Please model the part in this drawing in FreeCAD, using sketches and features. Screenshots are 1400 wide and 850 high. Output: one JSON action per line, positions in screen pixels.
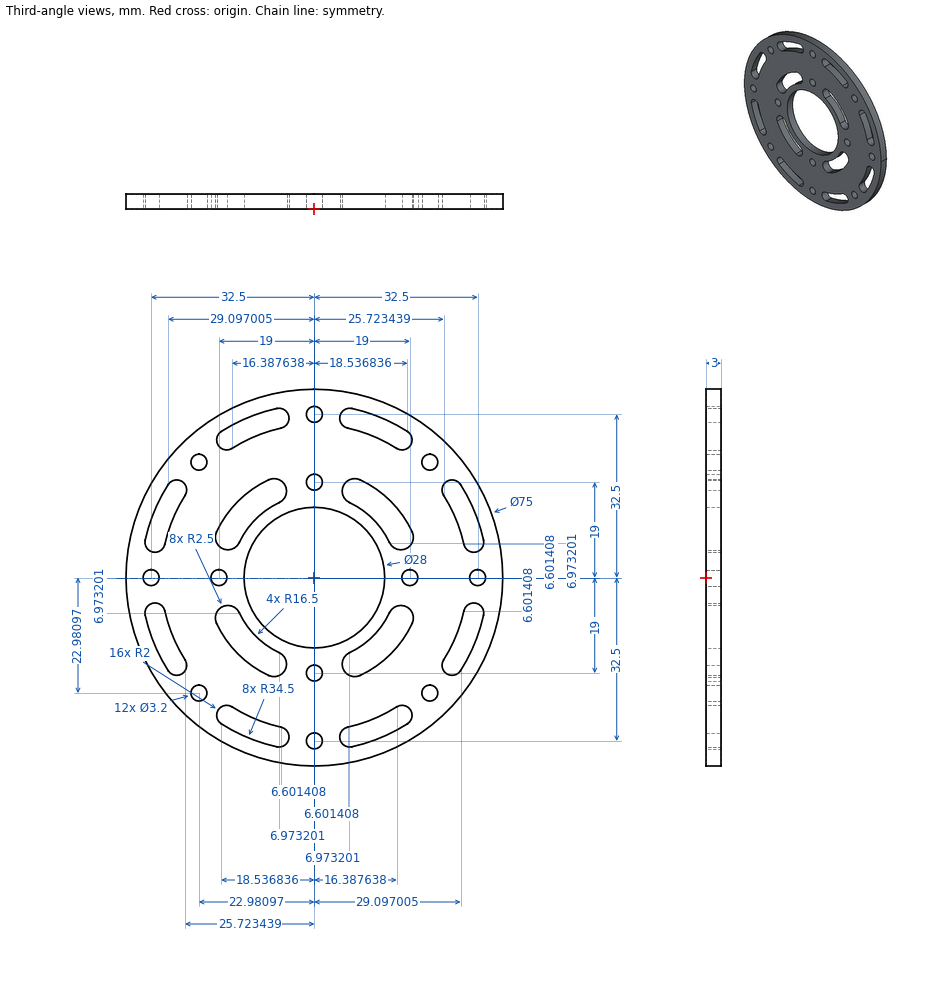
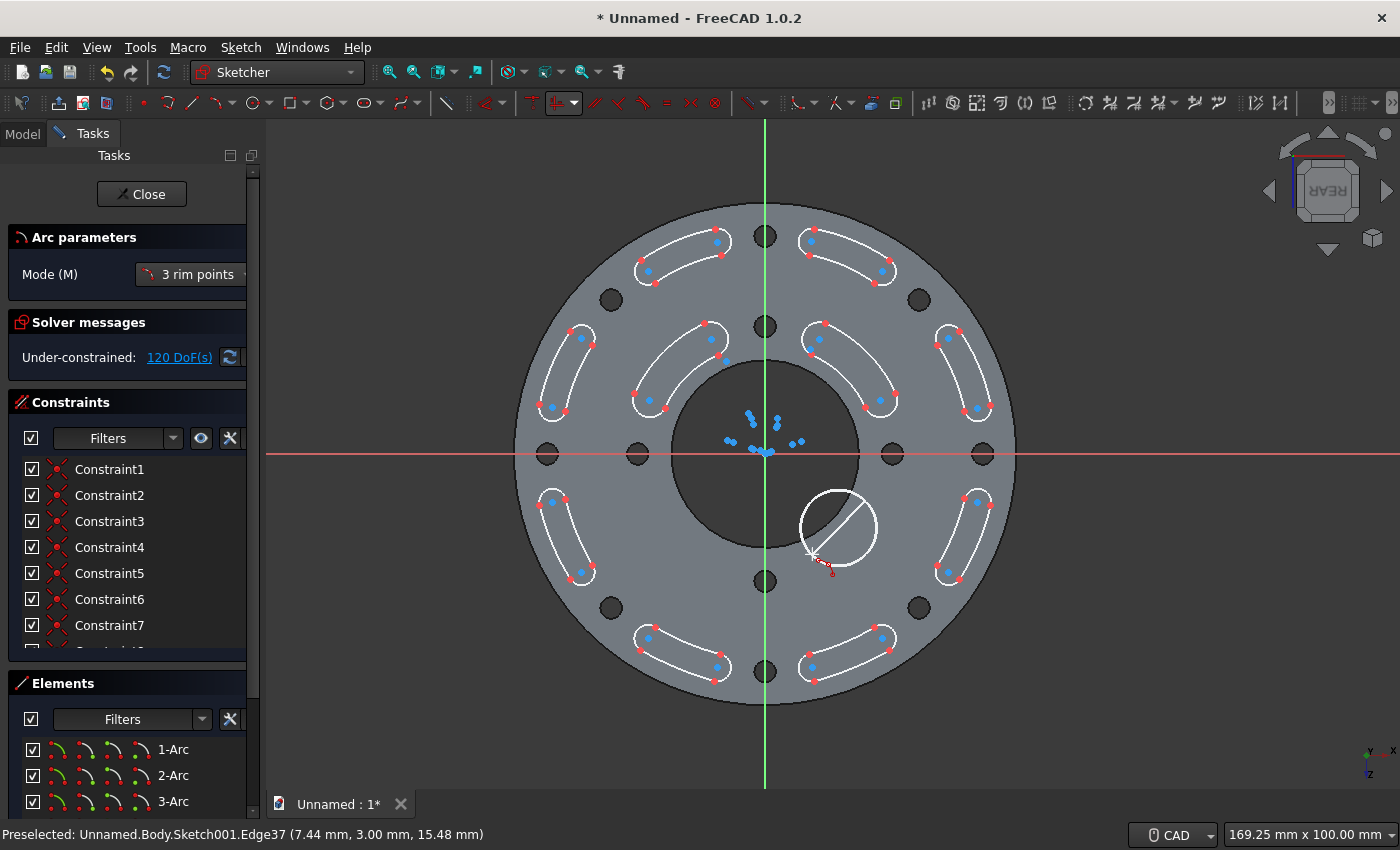
{"action": "scroll", "coordinate": [843, 532], "scroll_direction": "up", "scroll_amount": 5}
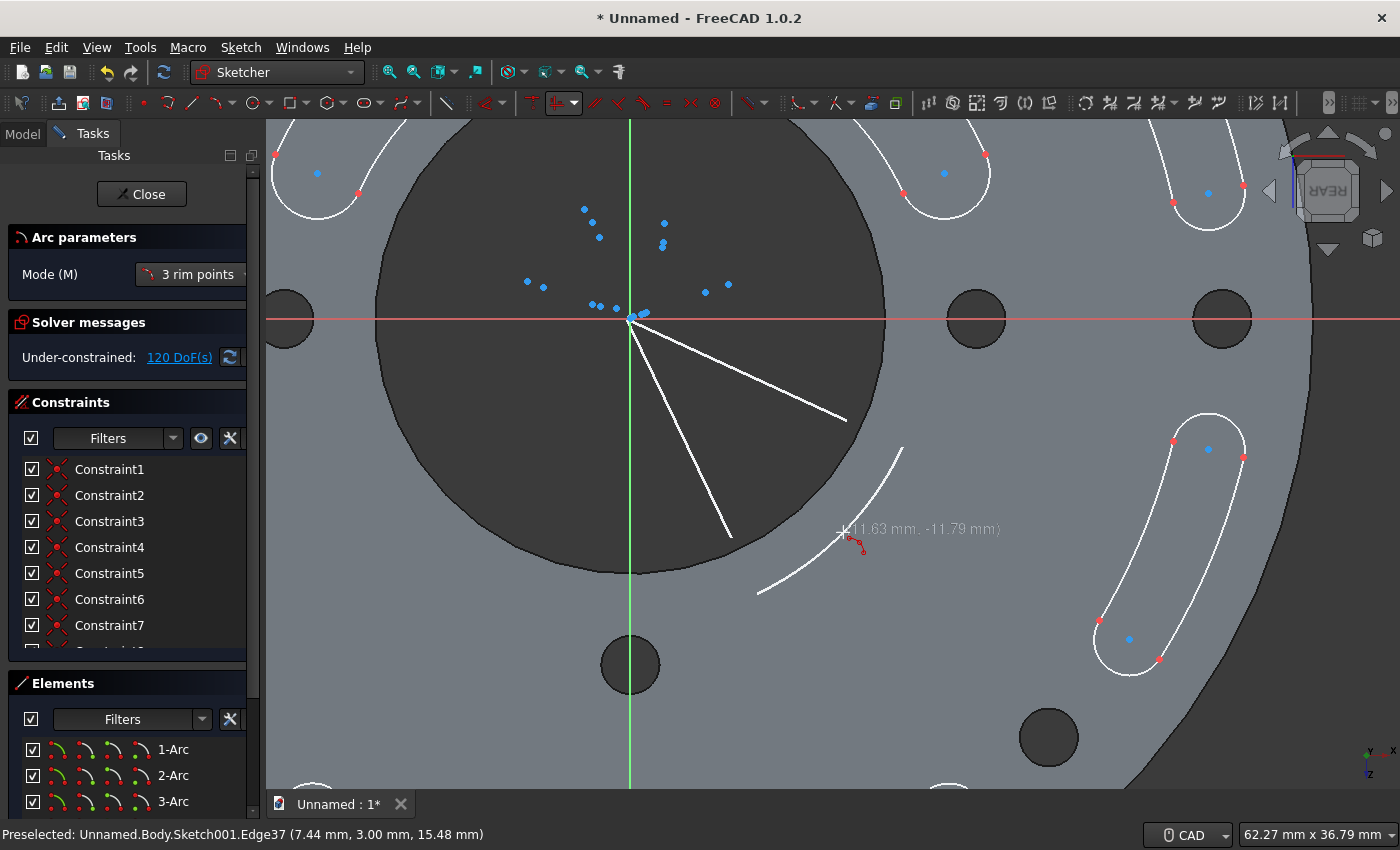
{"action": "left_click", "coordinate": [843, 531]}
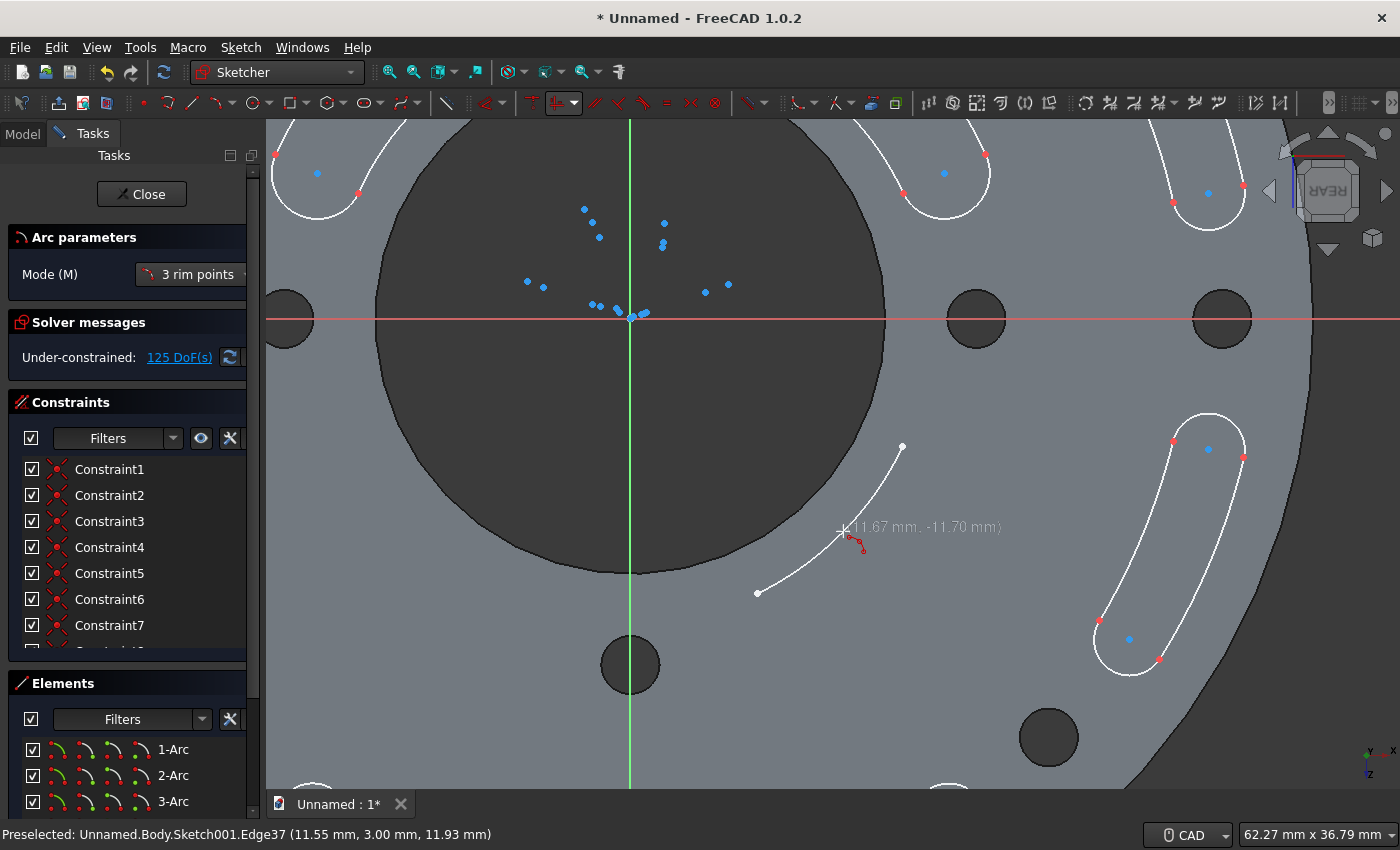
{"action": "left_click", "coordinate": [758, 593]}
{"action": "left_click", "coordinate": [796, 674]}
{"action": "left_click", "coordinate": [735, 652]}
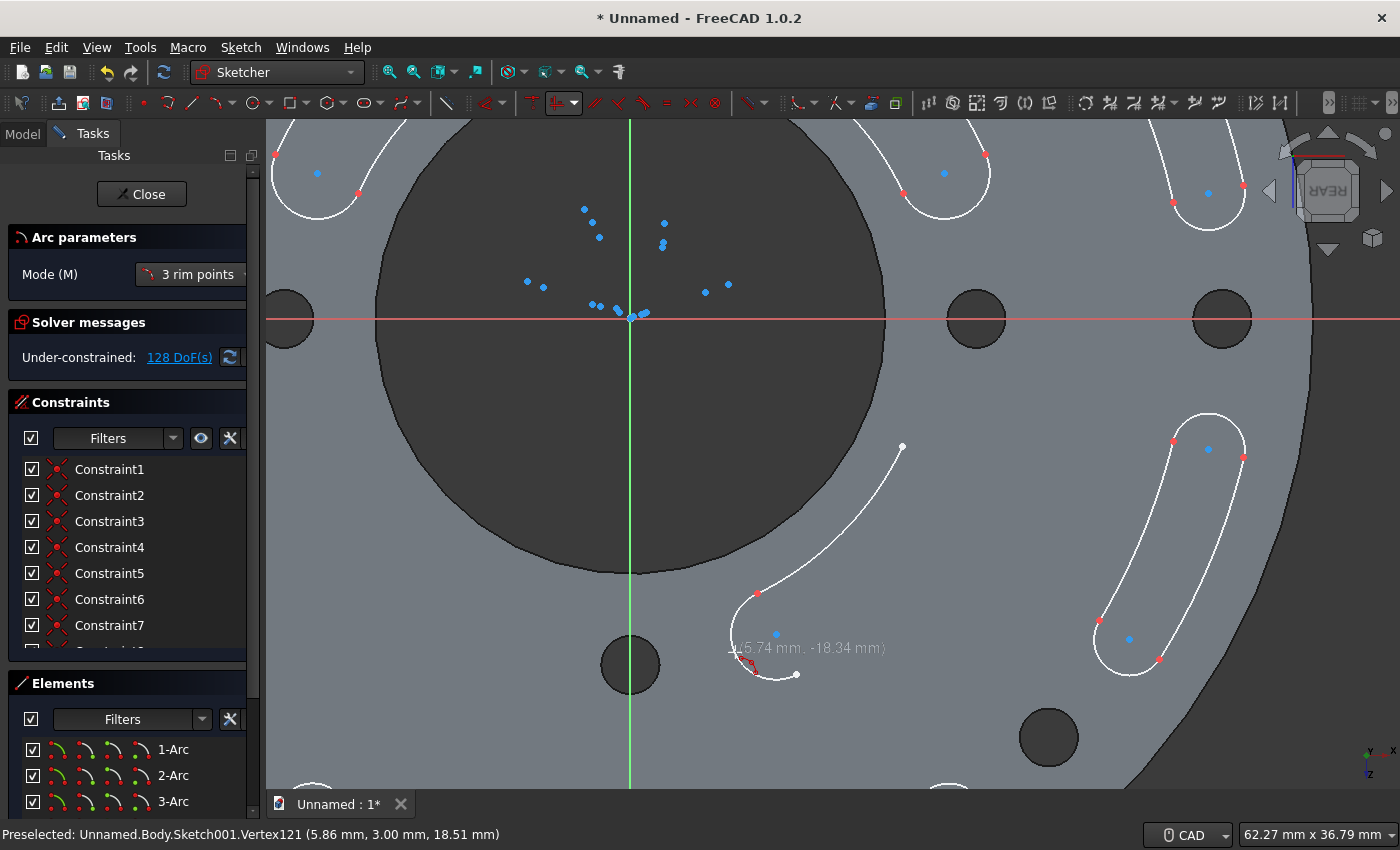
{"action": "left_click", "coordinate": [796, 675]}
{"action": "left_click", "coordinate": [985, 484]}
{"action": "left_click", "coordinate": [907, 596]}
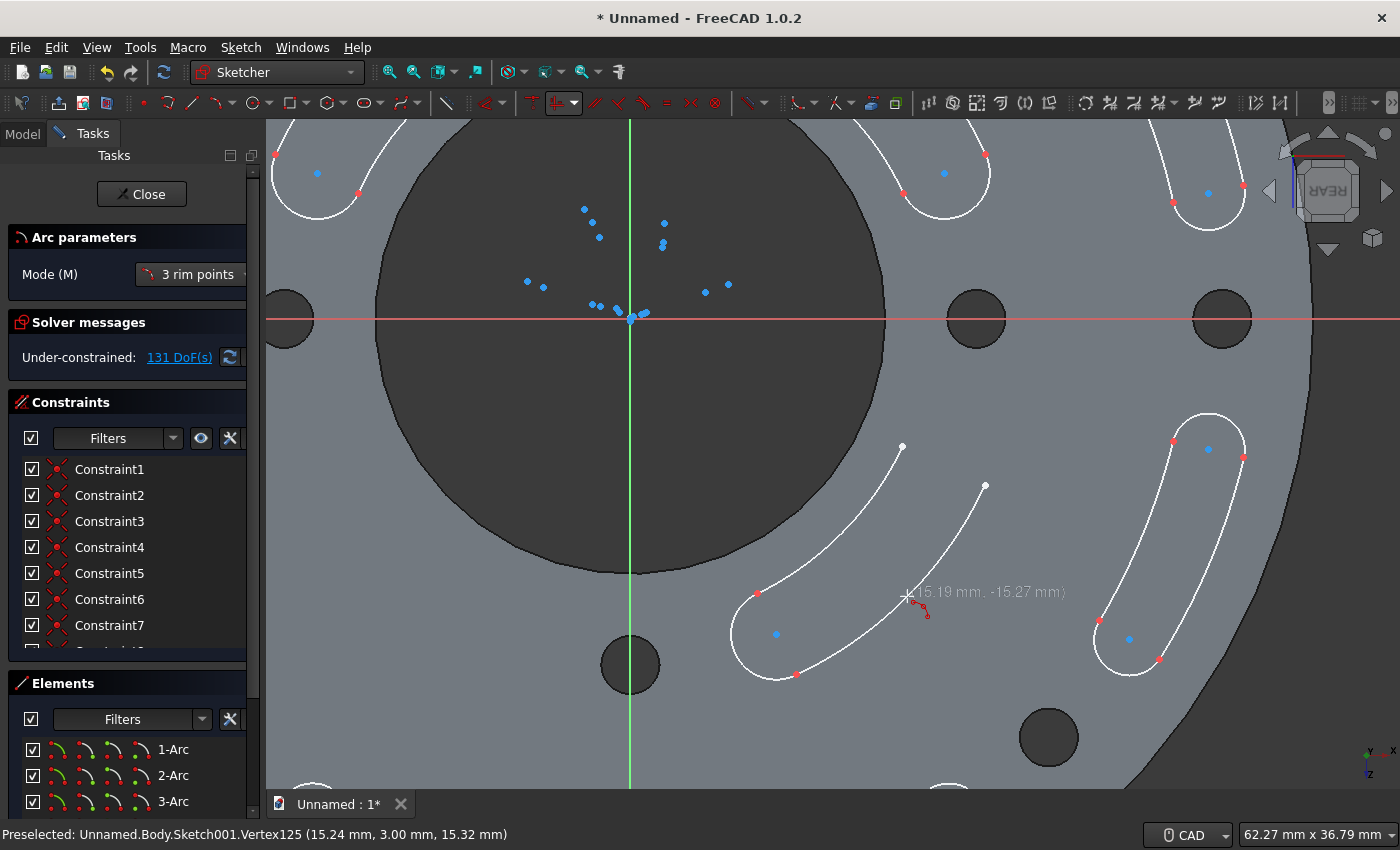
{"action": "left_click", "coordinate": [985, 485]}
{"action": "left_click", "coordinate": [903, 447]}
{"action": "left_click", "coordinate": [963, 424]}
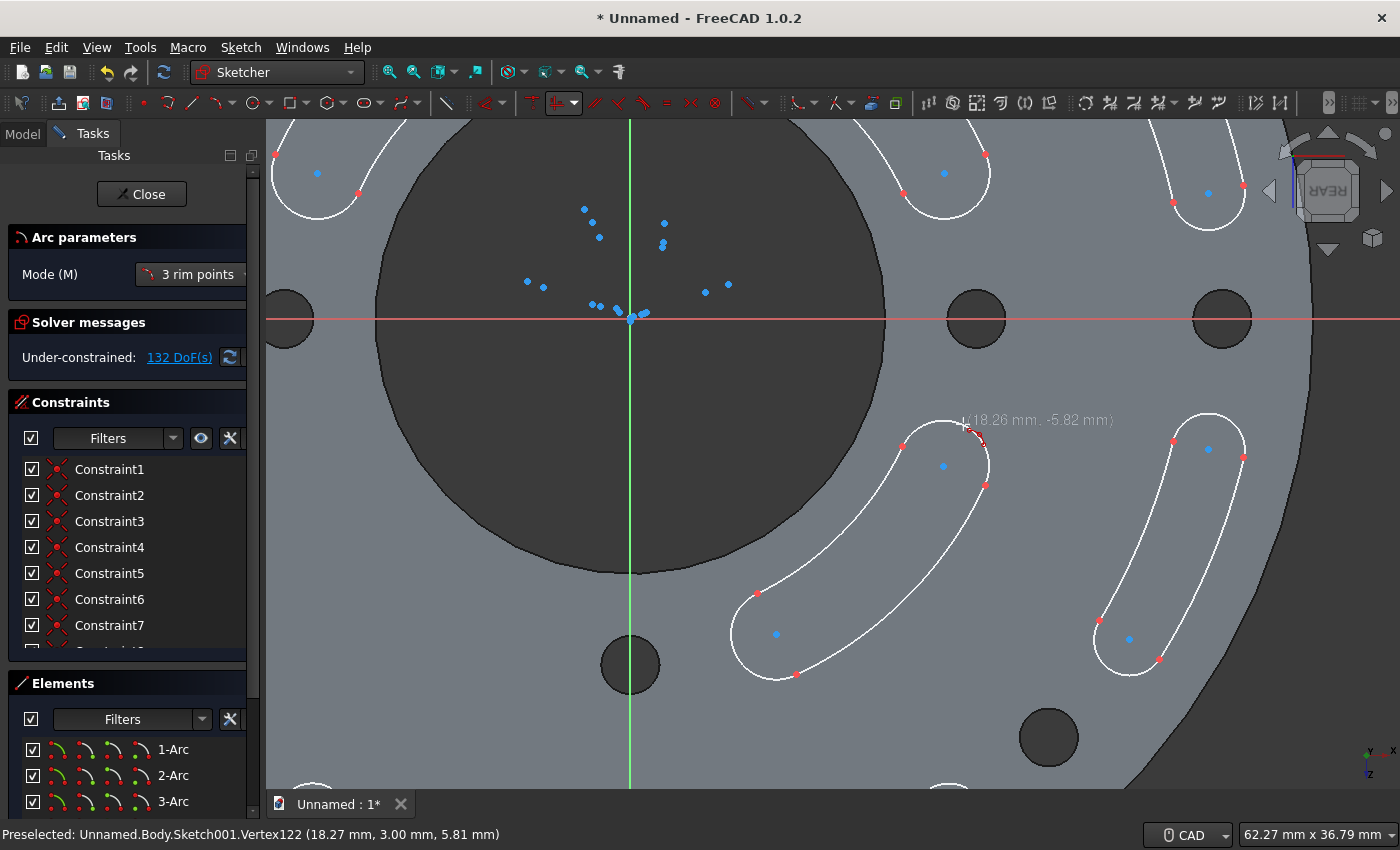
{"action": "left_click", "coordinate": [503, 591]}
{"action": "left_click", "coordinate": [358, 446]}
{"action": "left_click", "coordinate": [418, 531]}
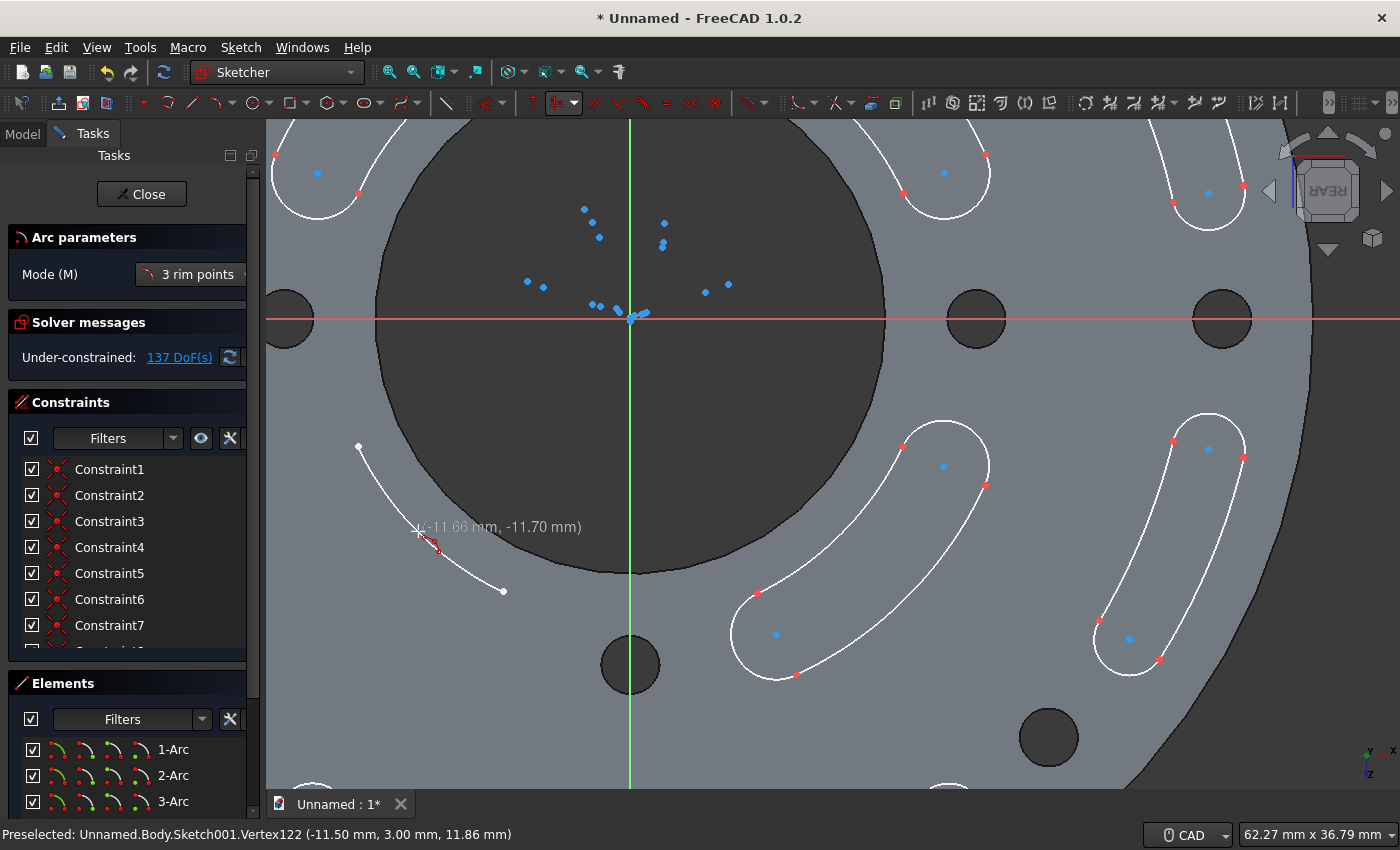
{"action": "left_click", "coordinate": [358, 447]}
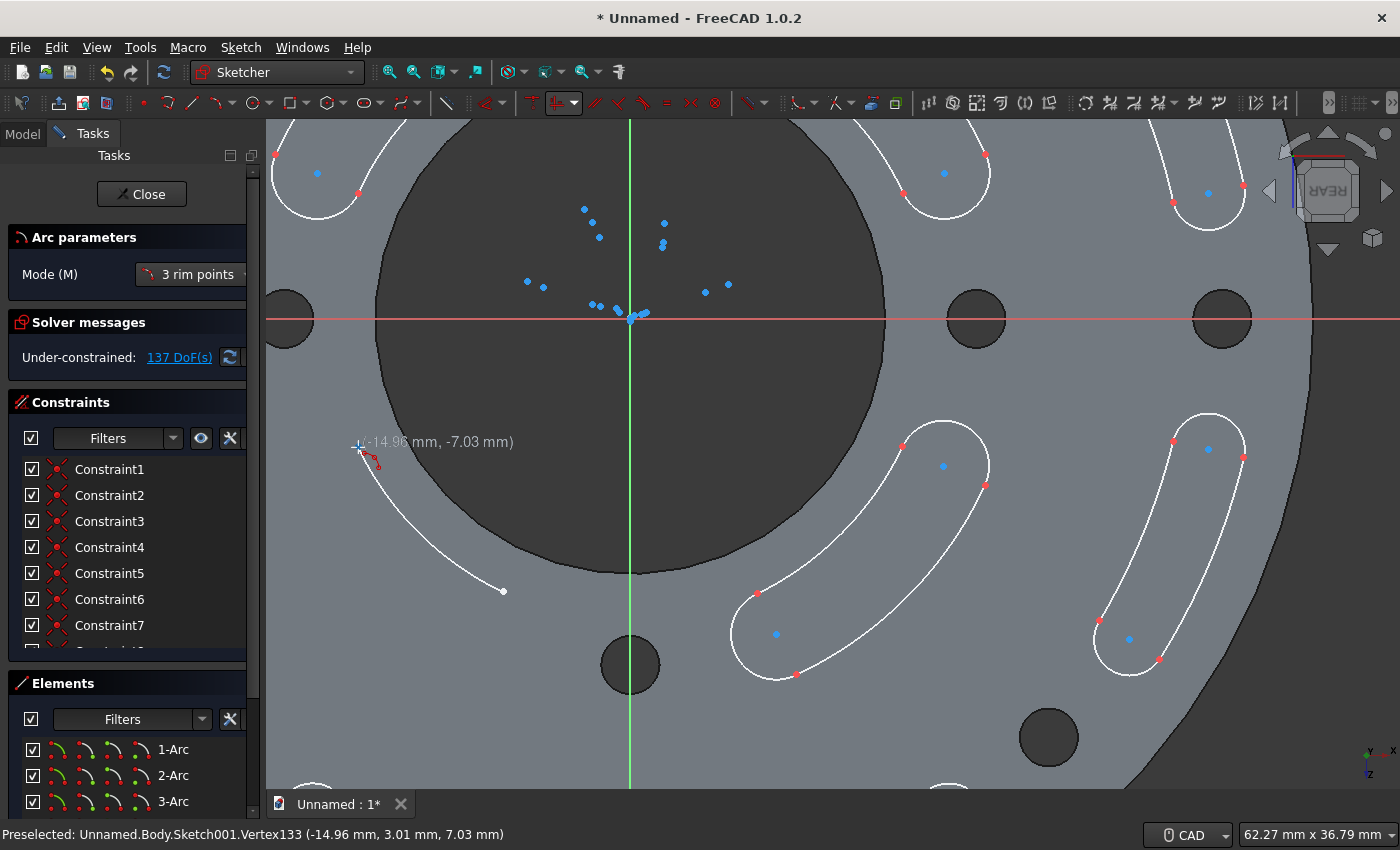
{"action": "scroll", "coordinate": [843, 533], "scroll_direction": "down", "scroll_amount": 5}